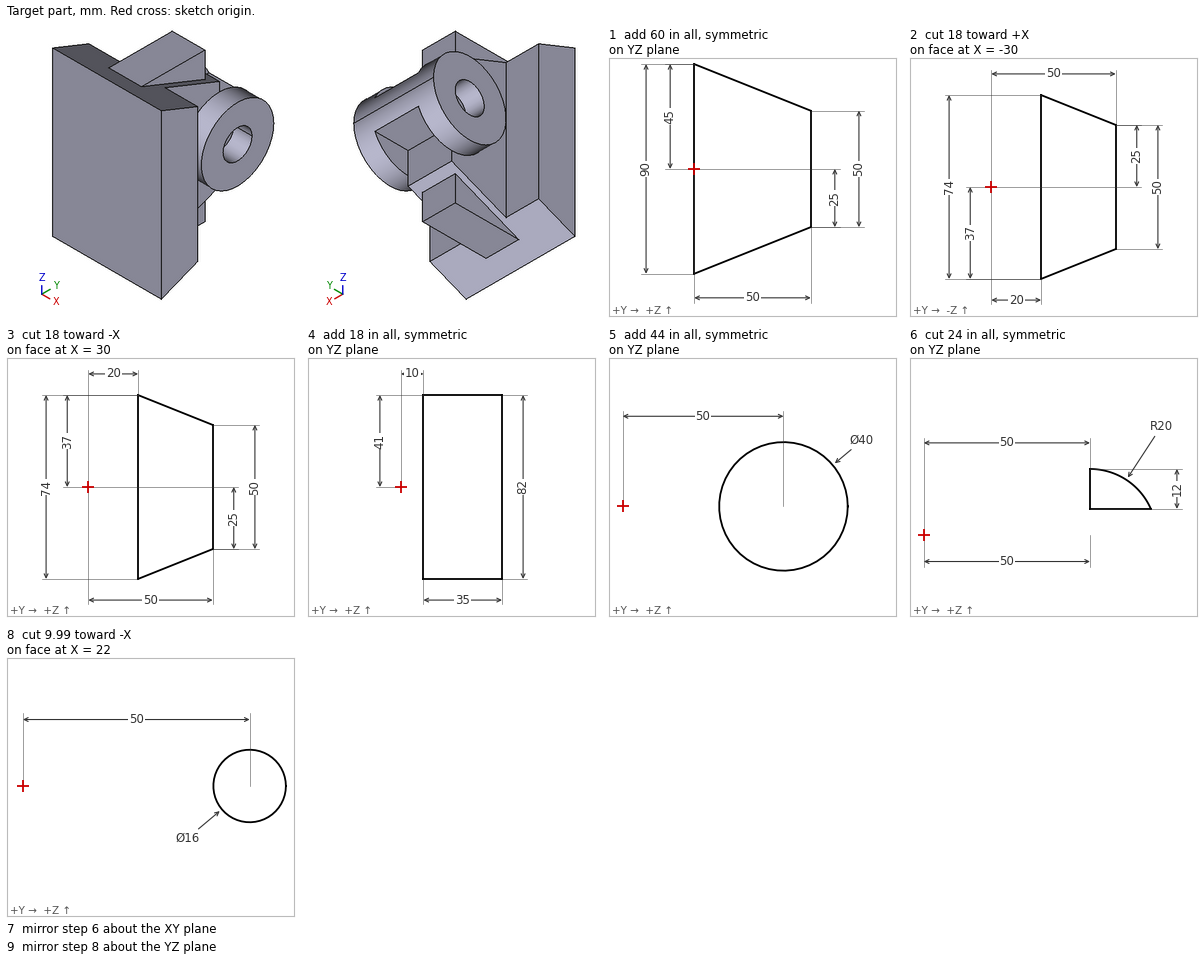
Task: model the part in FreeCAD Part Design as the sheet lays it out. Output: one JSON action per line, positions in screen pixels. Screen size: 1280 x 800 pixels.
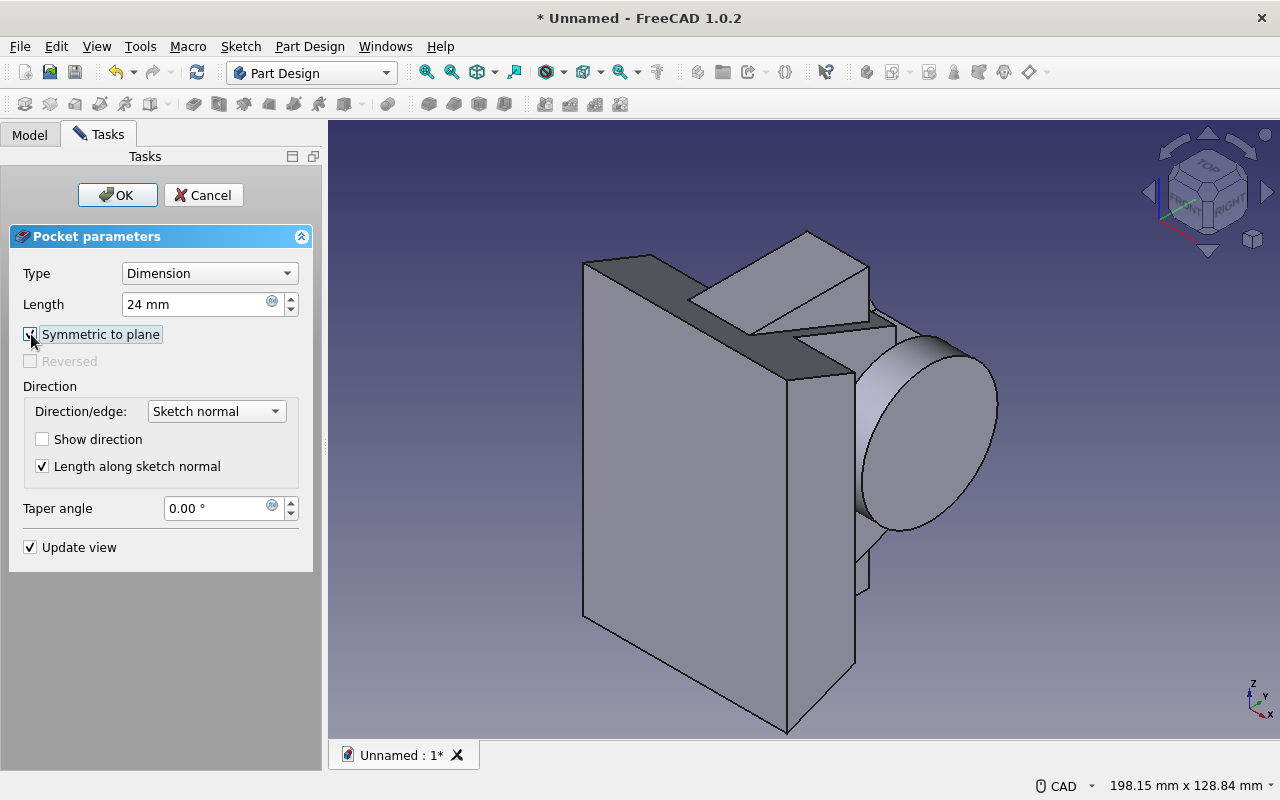
{"action": "left_click", "coordinate": [118, 195]}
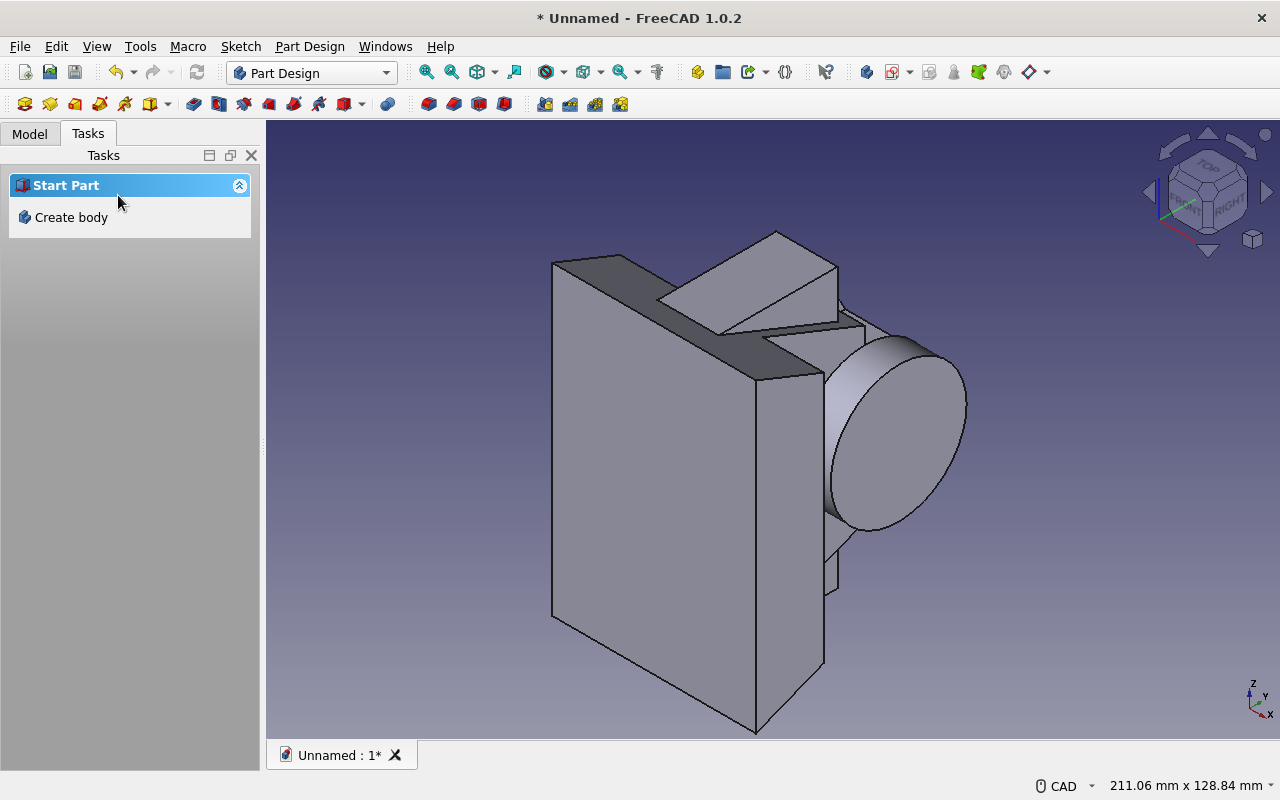
{"action": "left_click", "coordinate": [30, 134]}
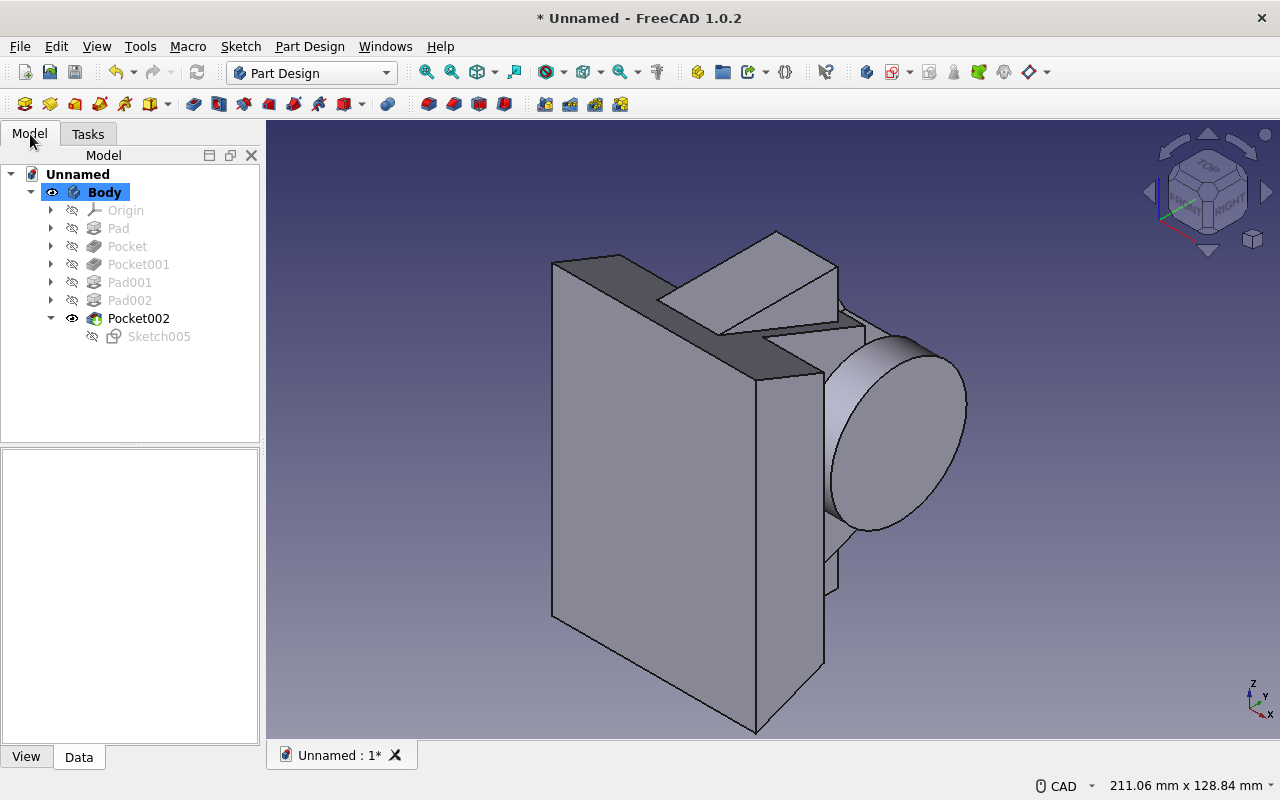
{"action": "left_click", "coordinate": [117, 318]}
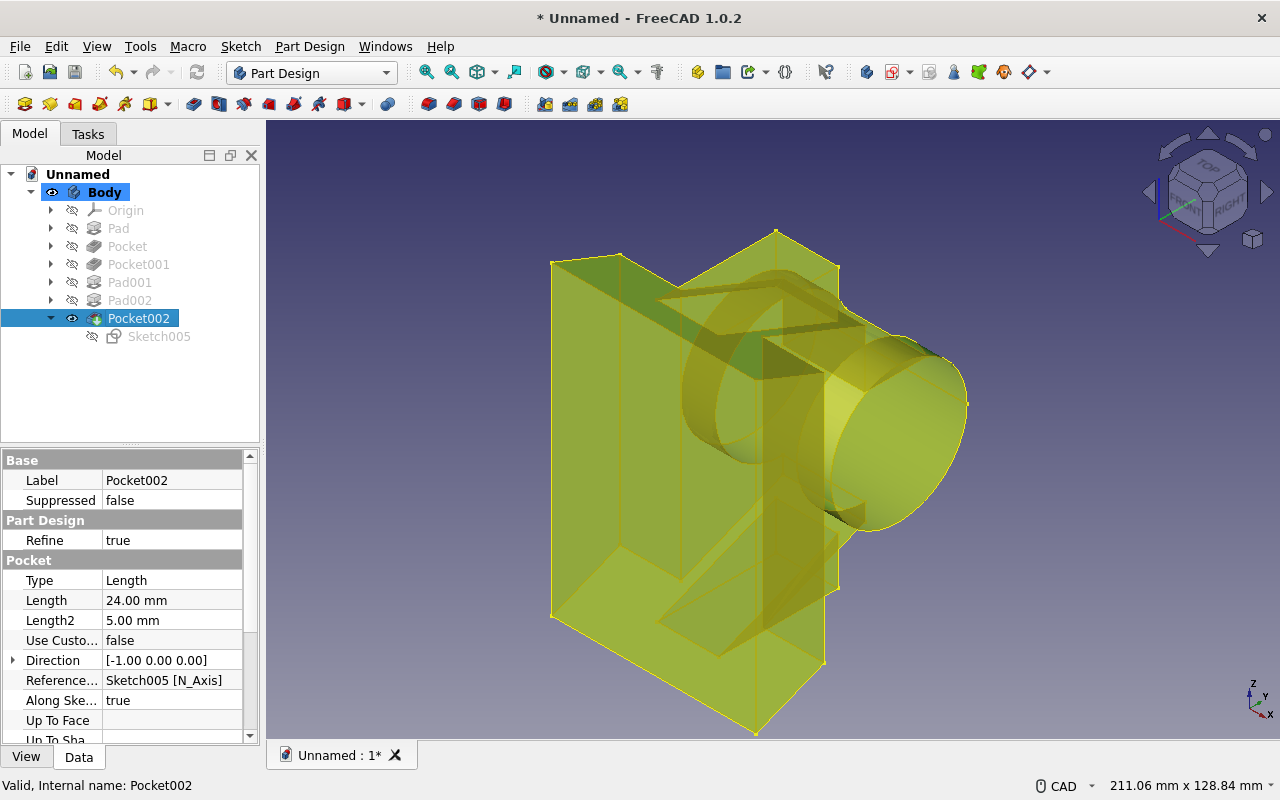
{"action": "left_click", "coordinate": [545, 104]}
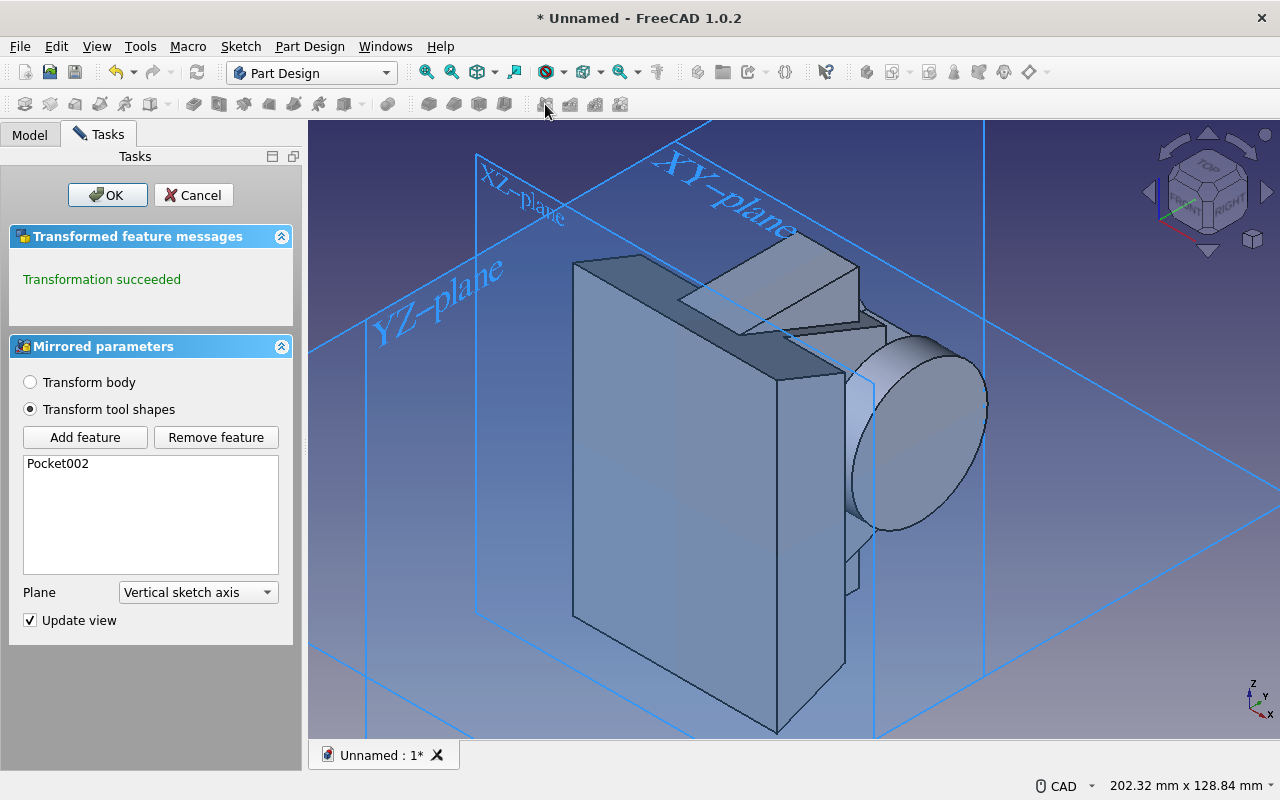
{"action": "left_click", "coordinate": [199, 592]}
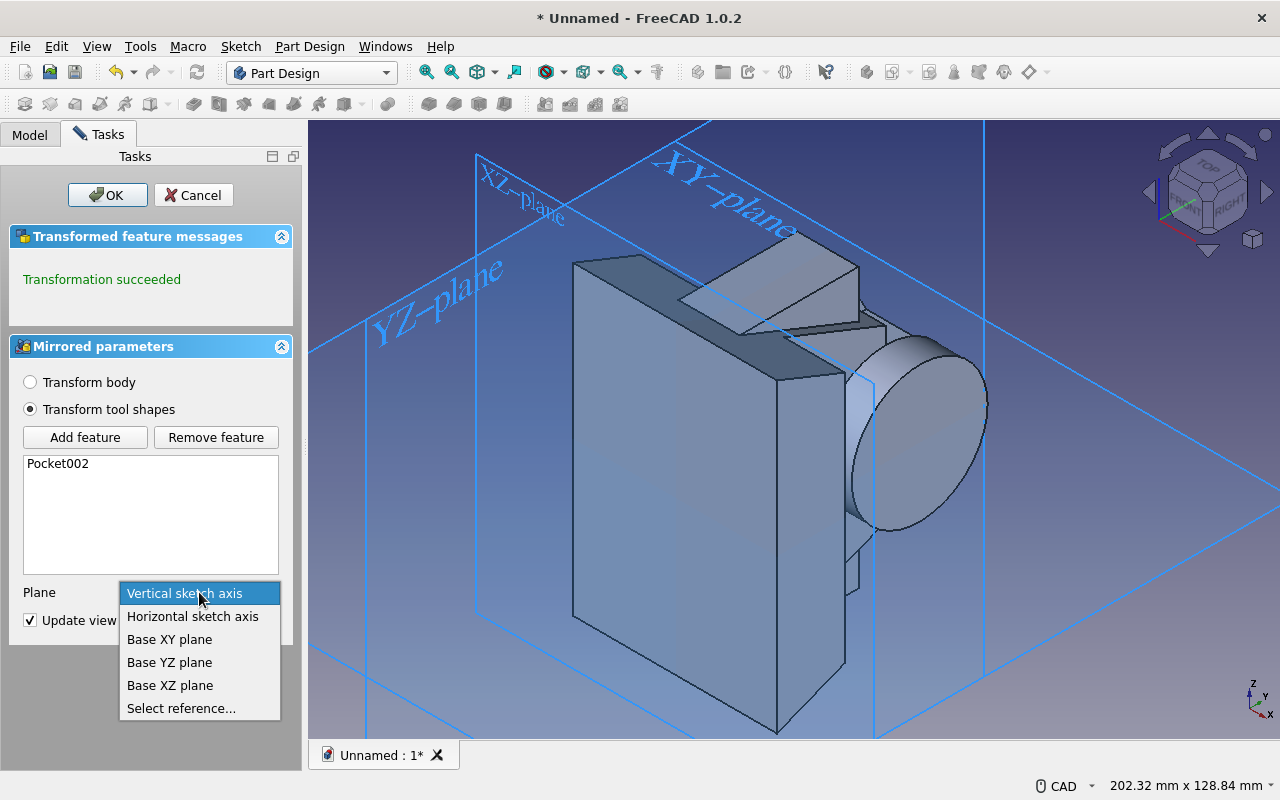
{"action": "left_click", "coordinate": [198, 640]}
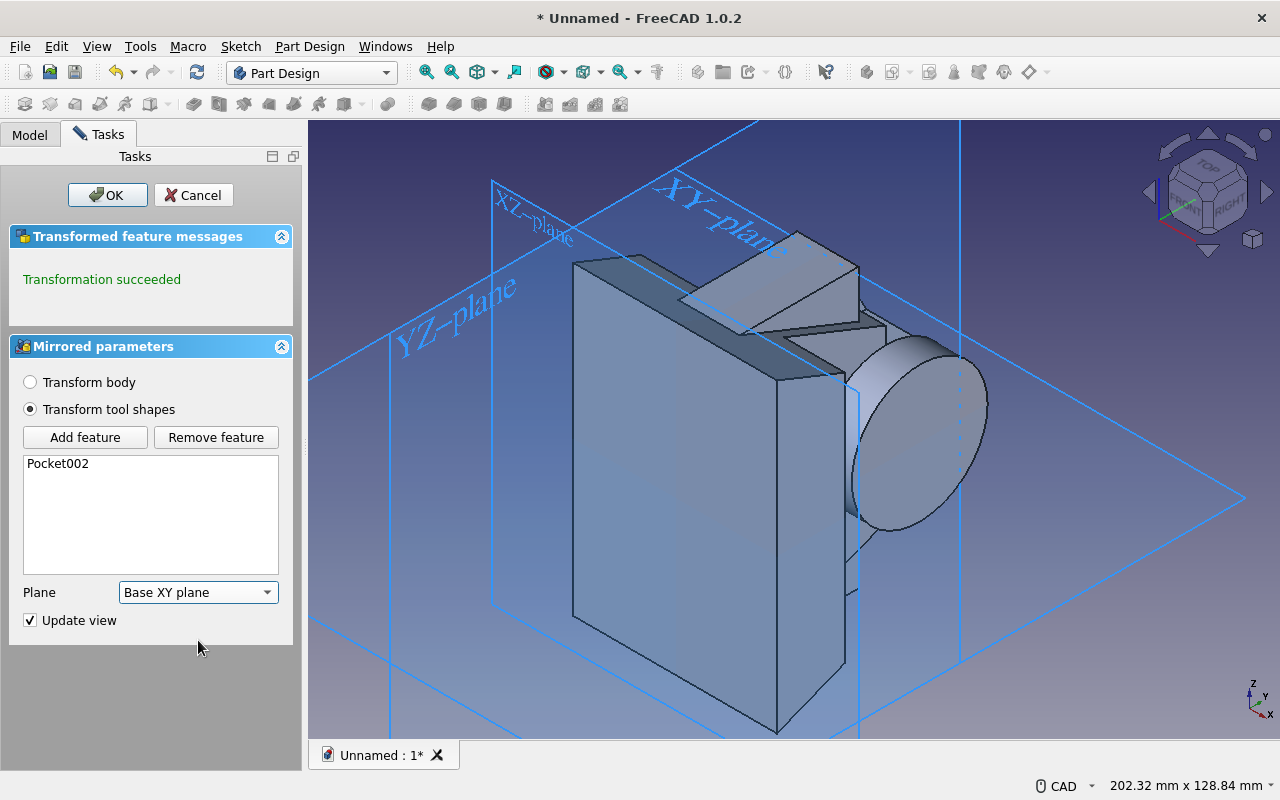
{"action": "left_click", "coordinate": [108, 195]}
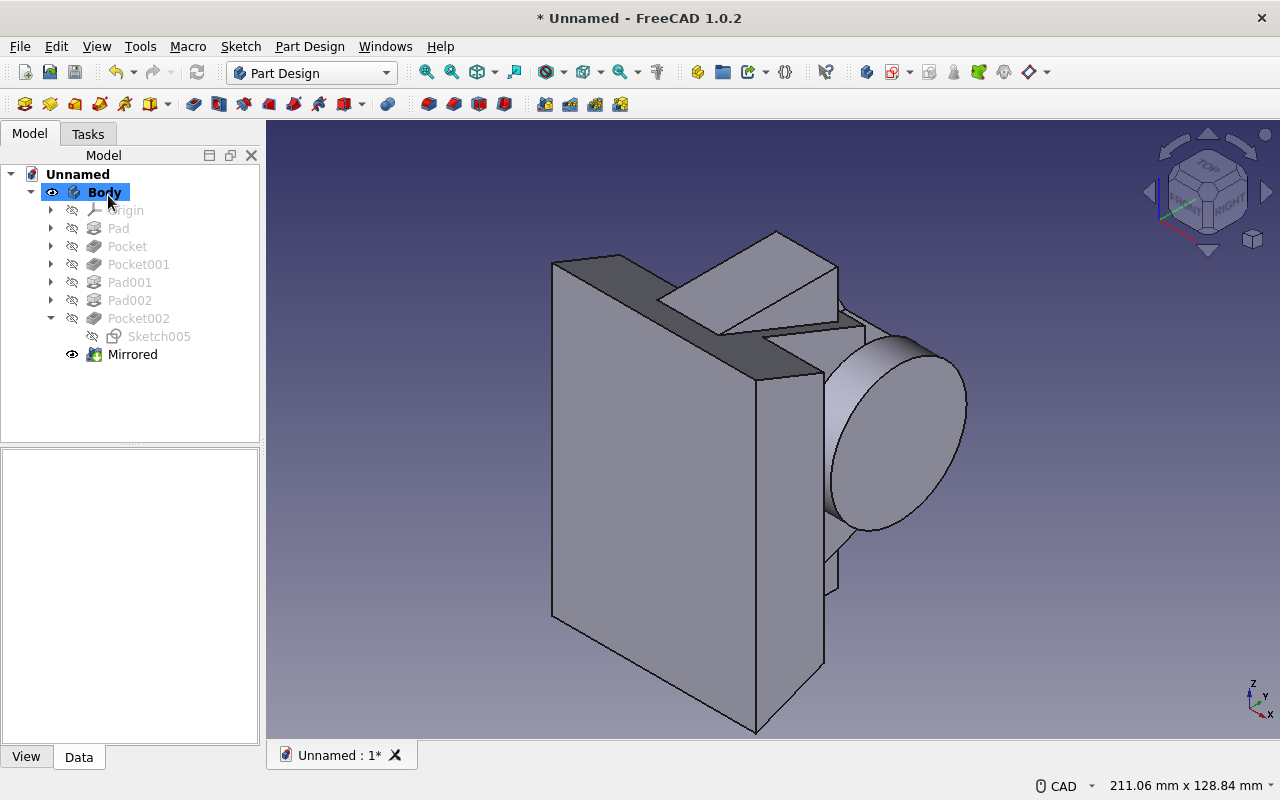
{"action": "left_click", "coordinate": [899, 442]}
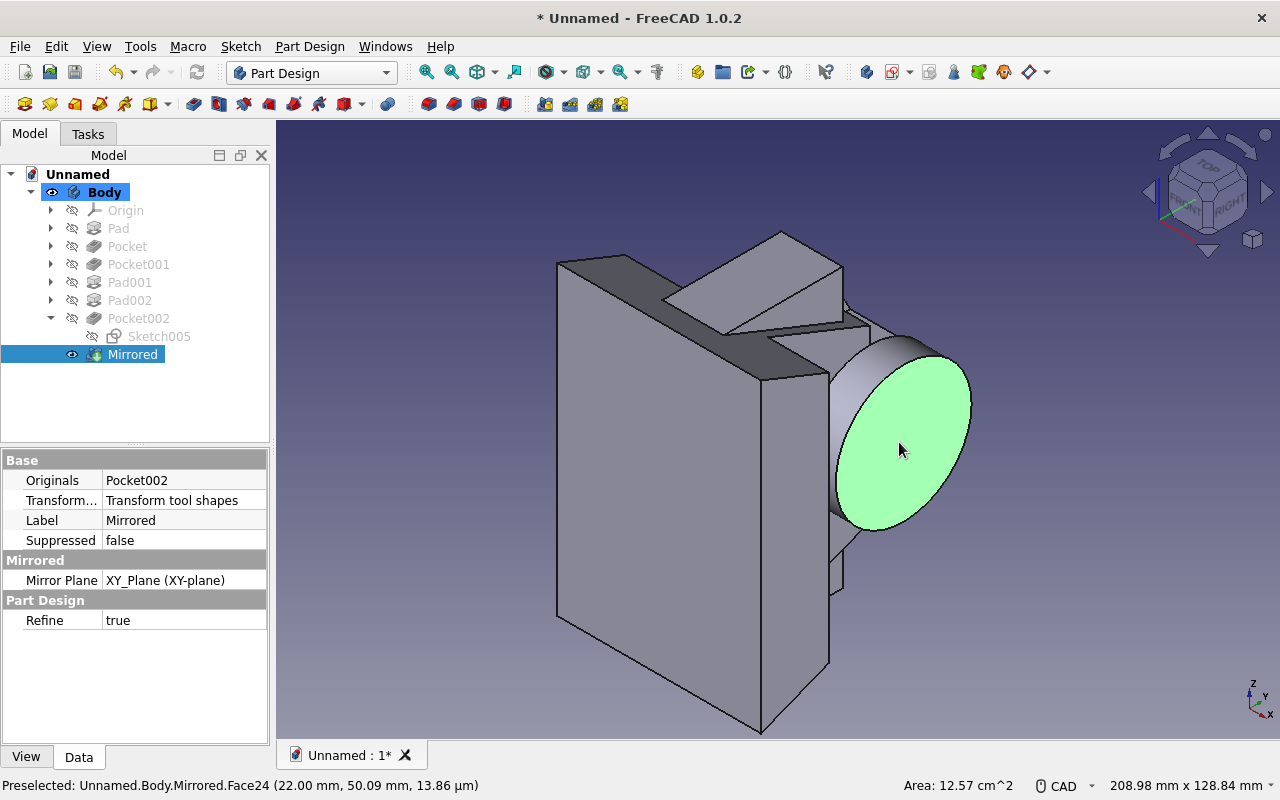
{"action": "left_click", "coordinate": [892, 72]}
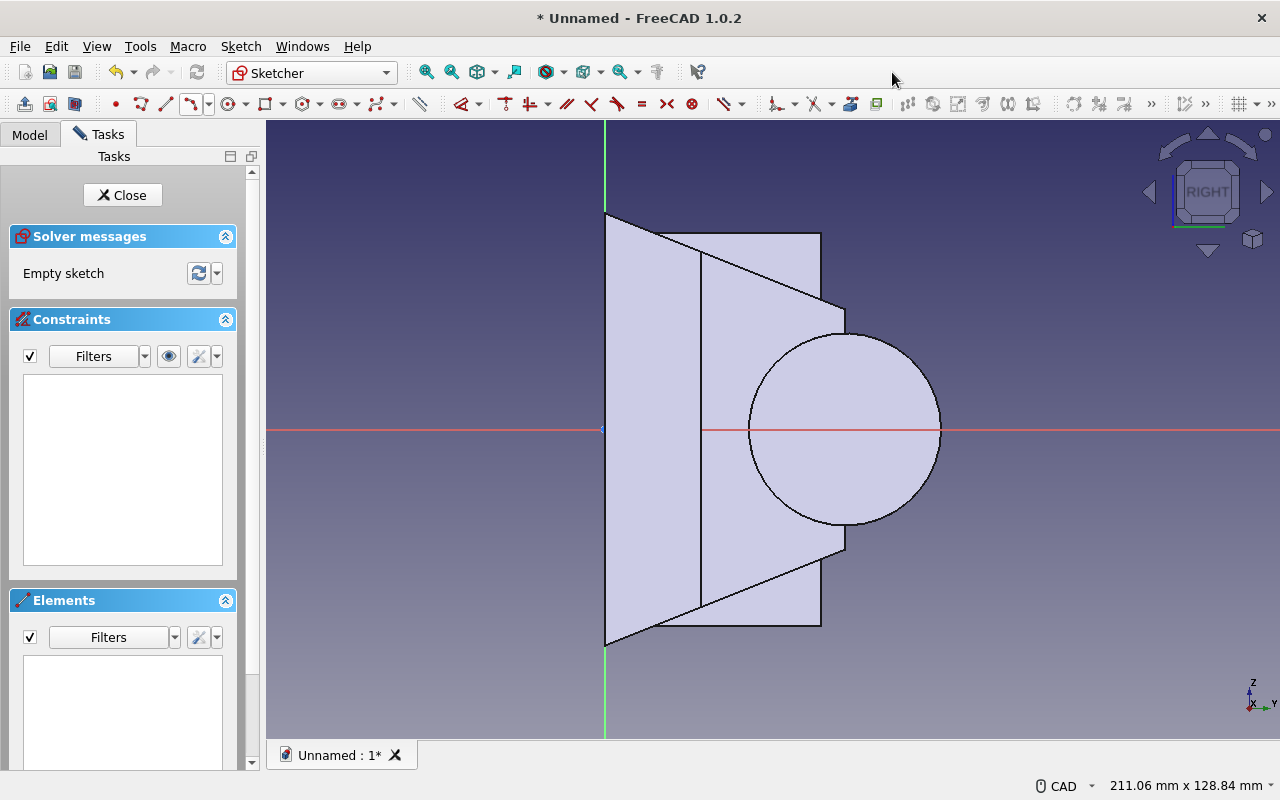
{"action": "scroll", "coordinate": [881, 430], "scroll_direction": "up", "scroll_amount": 8}